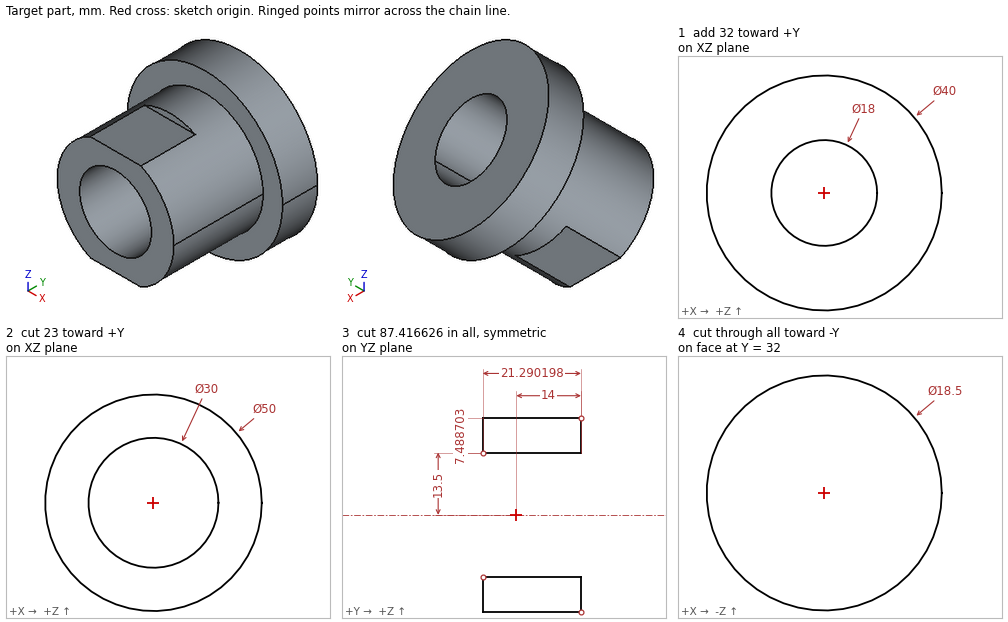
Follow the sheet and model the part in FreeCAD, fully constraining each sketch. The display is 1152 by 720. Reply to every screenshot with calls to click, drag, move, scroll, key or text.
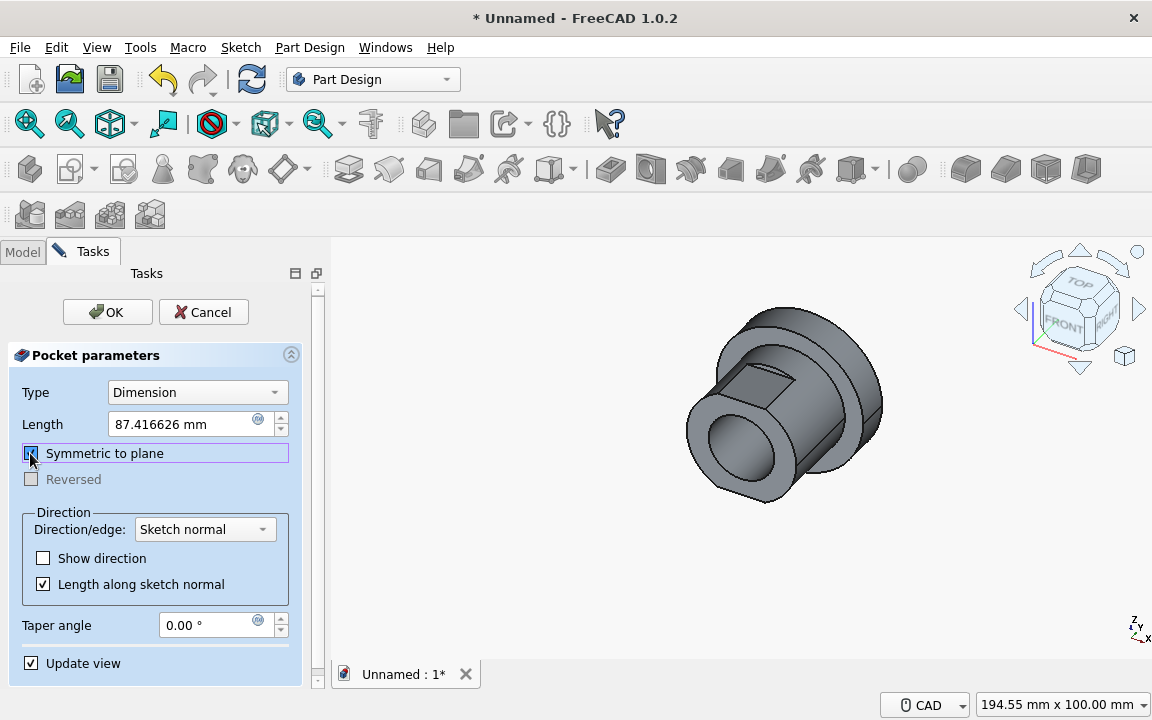
click(108, 312)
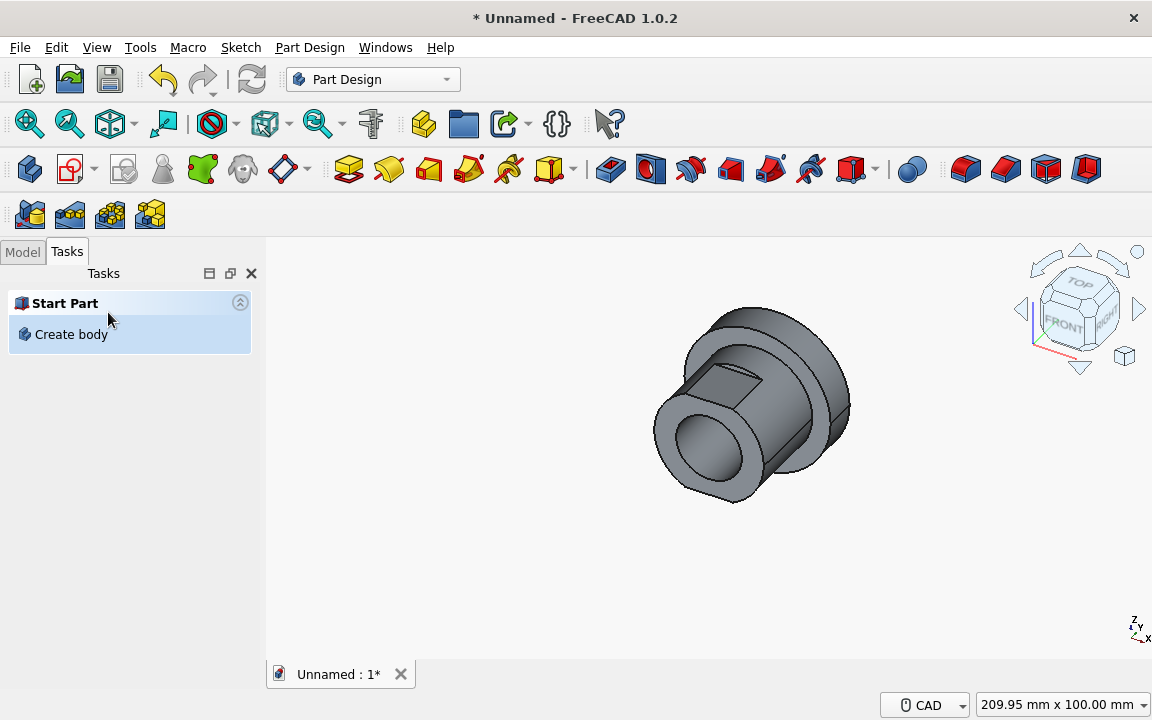
key(4)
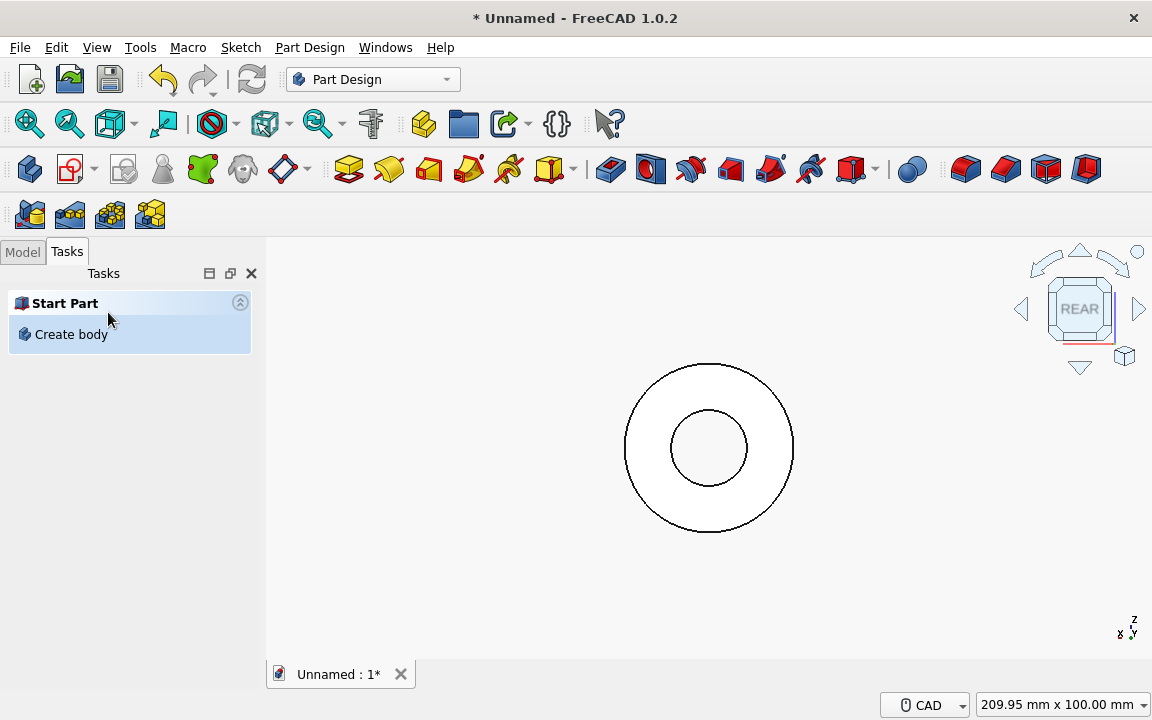
click(30, 124)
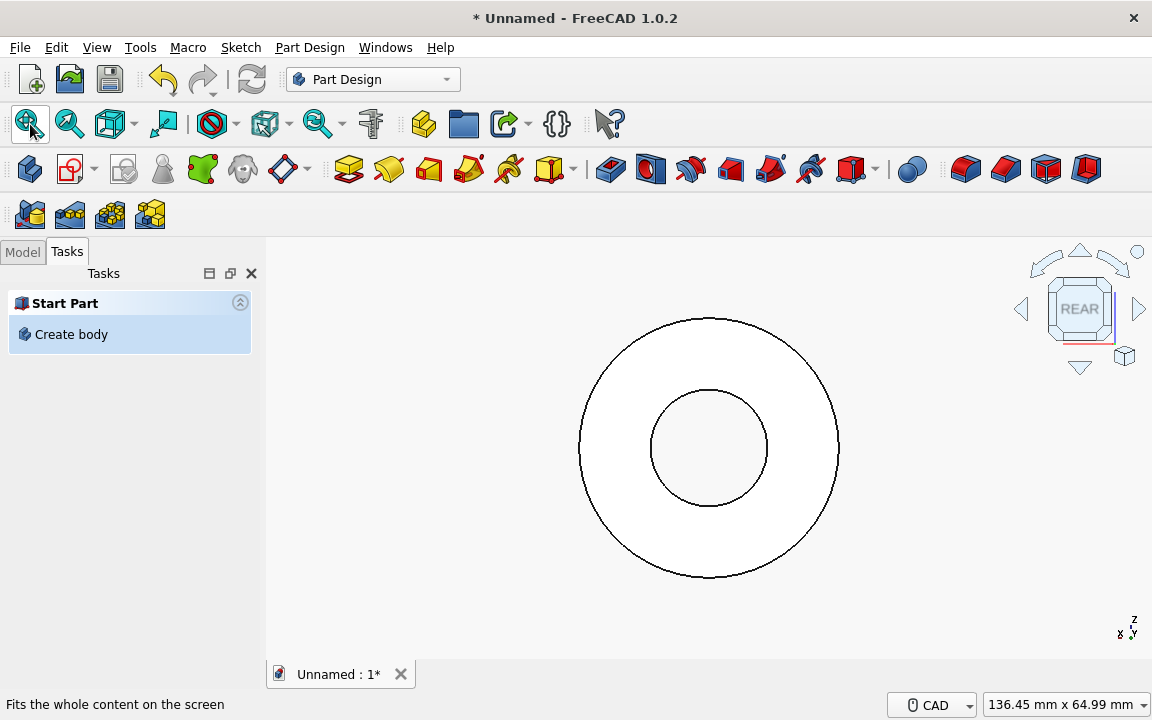
click(783, 521)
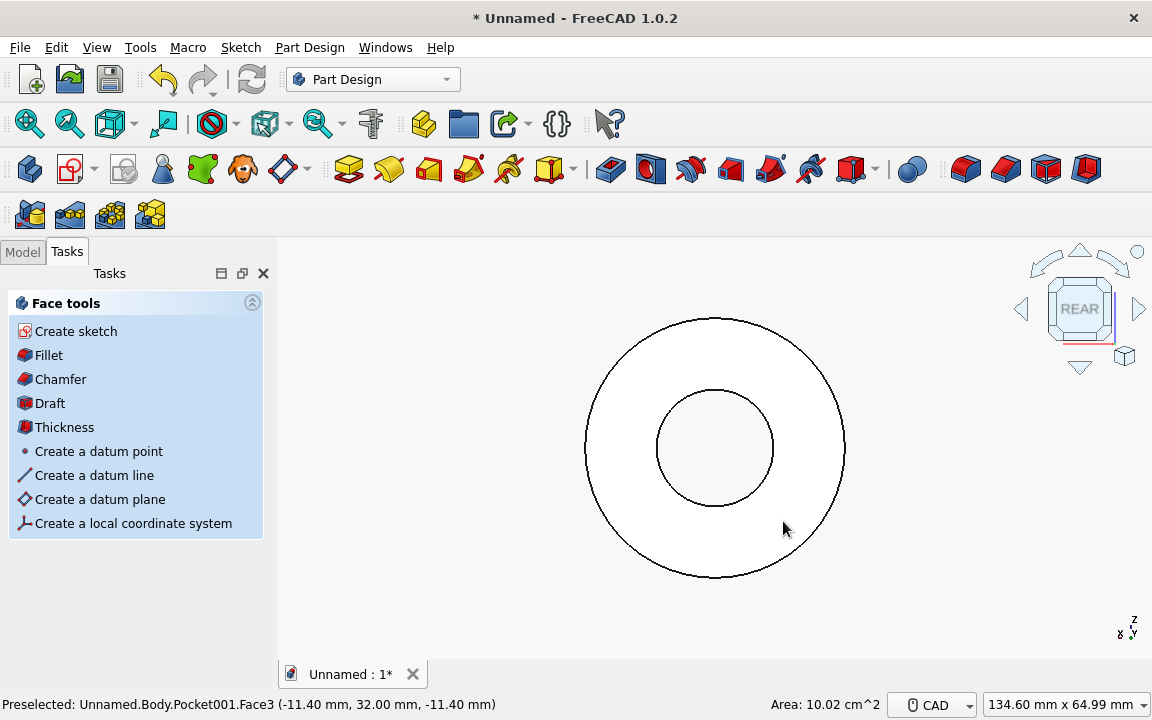
click(70, 170)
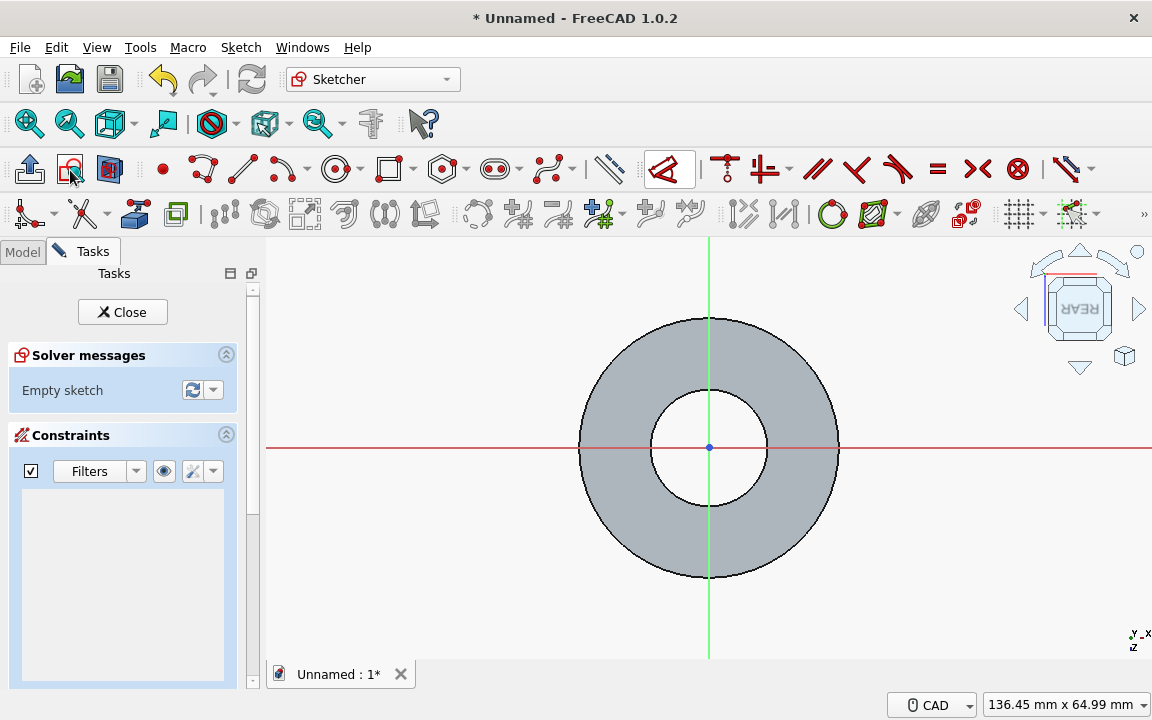
scroll(765, 448, up, 4)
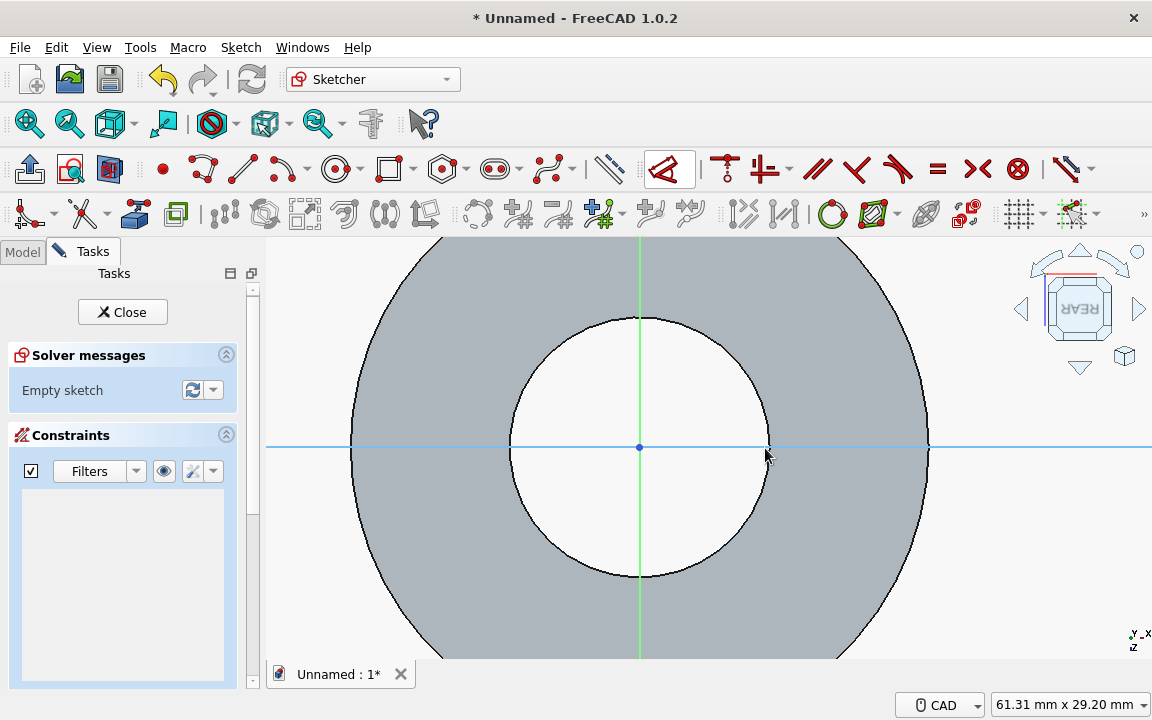
click(336, 170)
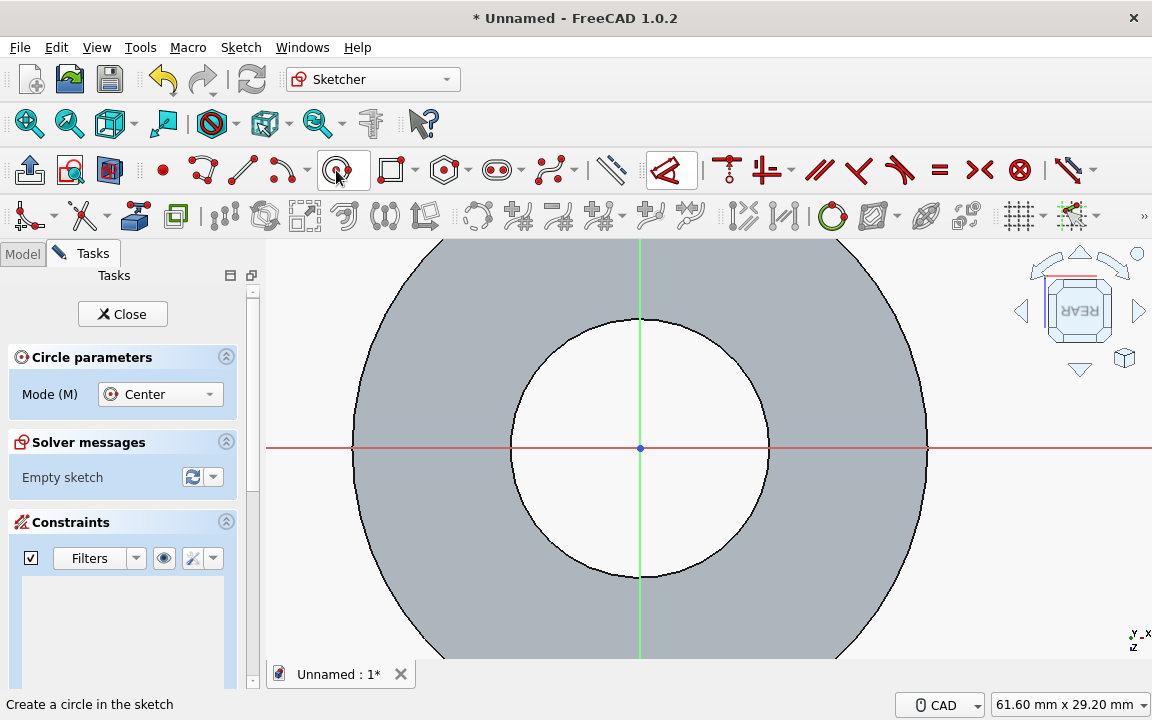
click(640, 448)
click(734, 354)
key(Escape)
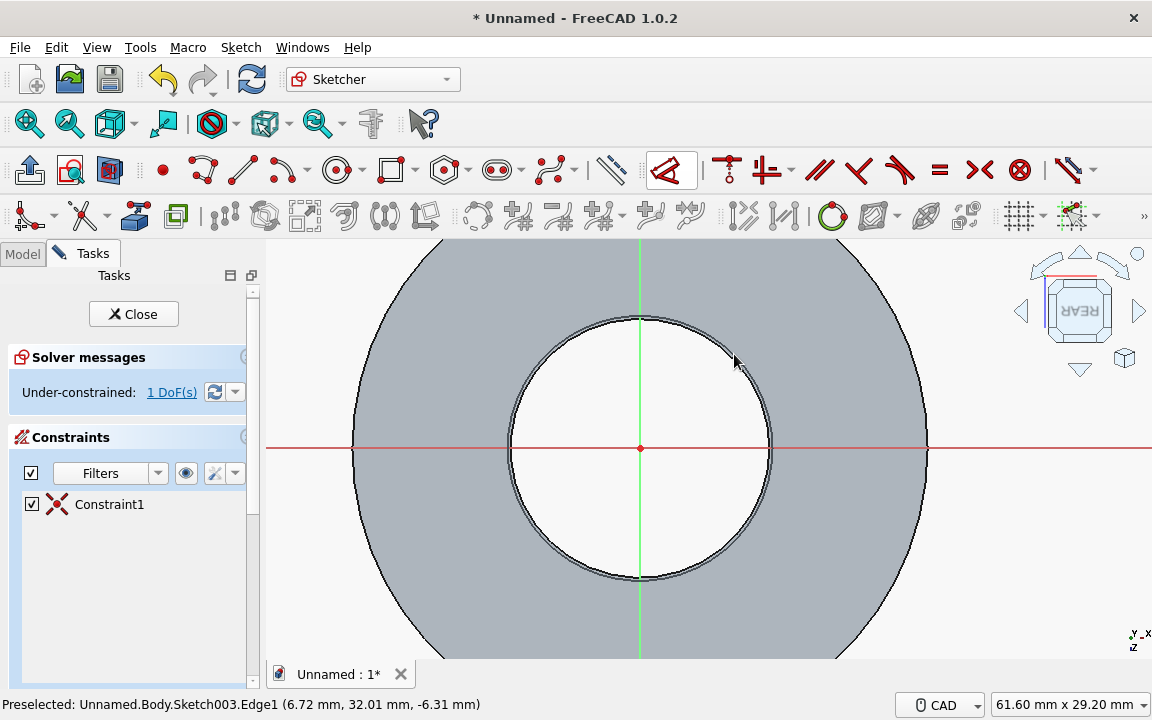
click(733, 354)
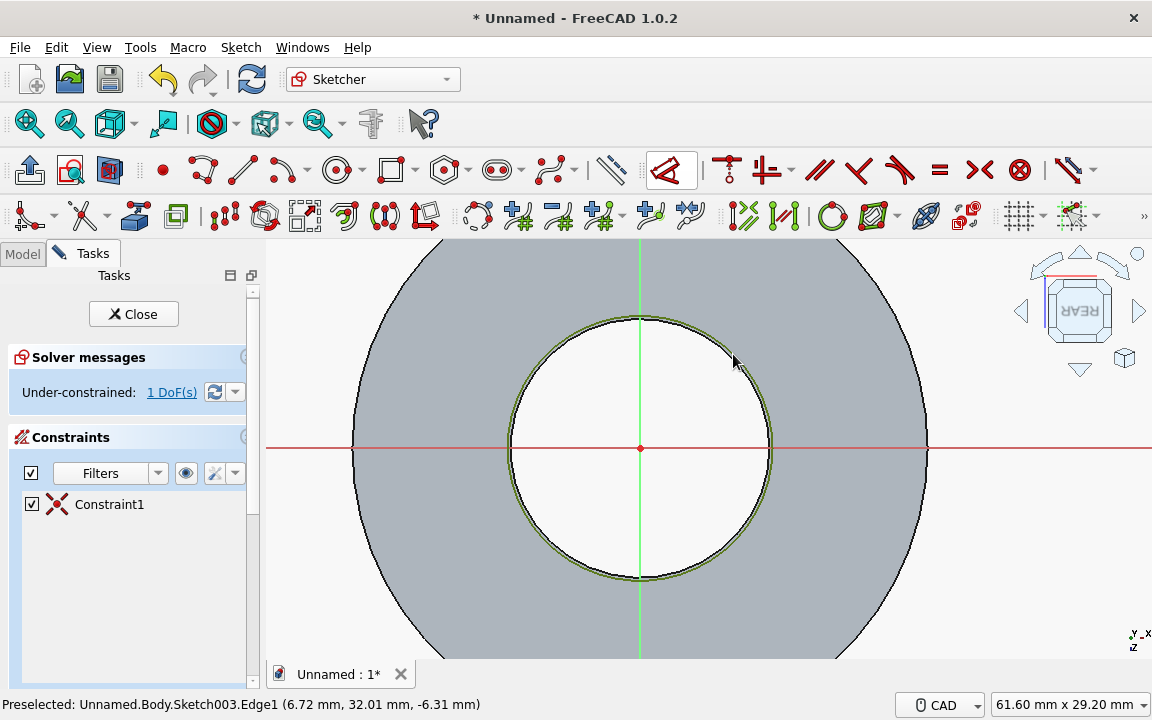
click(692, 170)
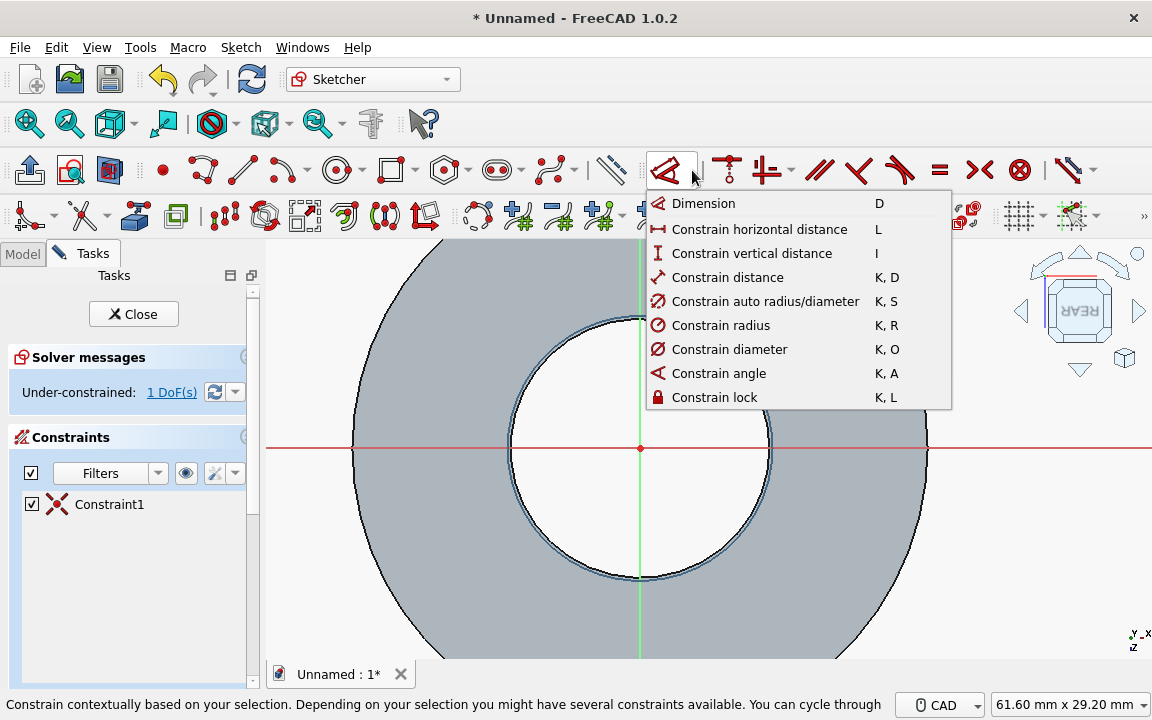
click(799, 349)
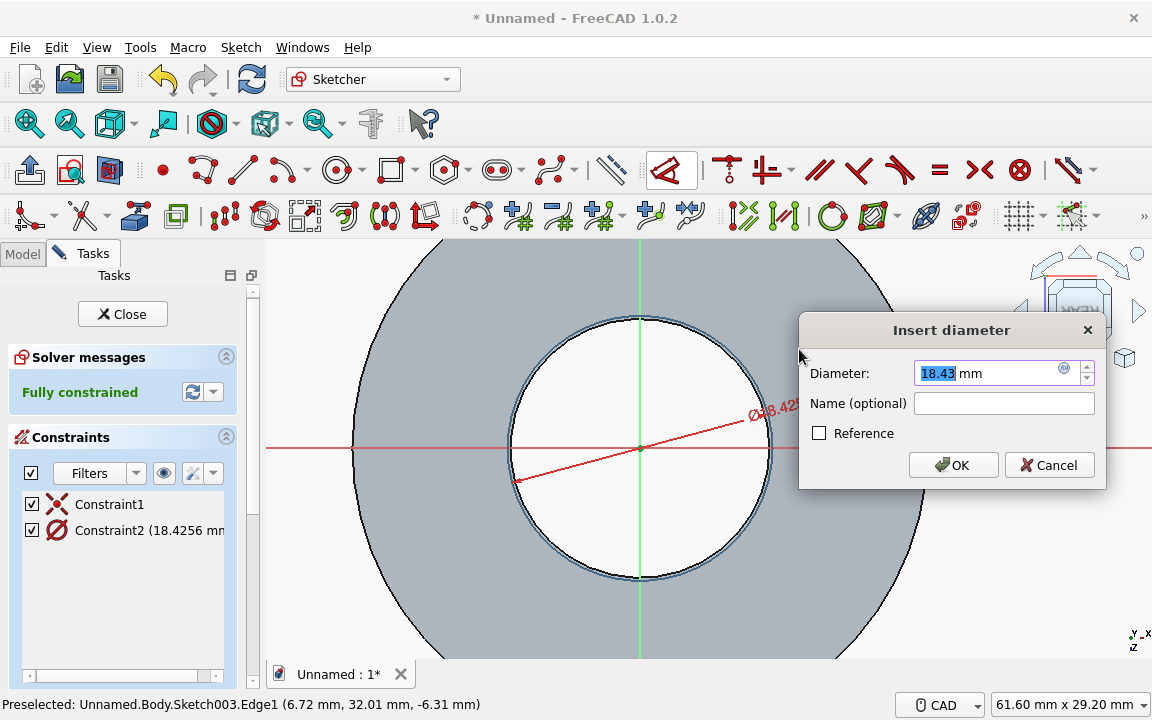
text(18.5)
key(Return)